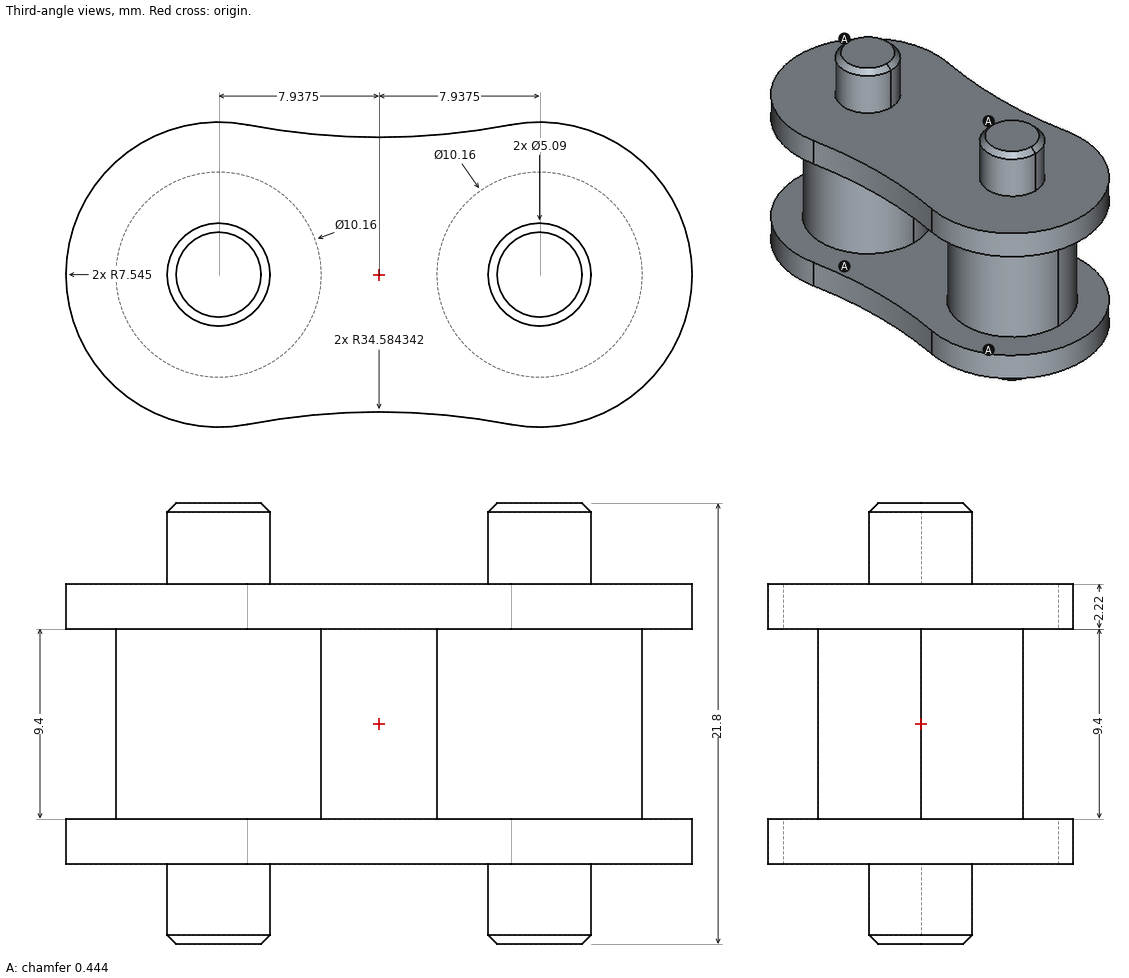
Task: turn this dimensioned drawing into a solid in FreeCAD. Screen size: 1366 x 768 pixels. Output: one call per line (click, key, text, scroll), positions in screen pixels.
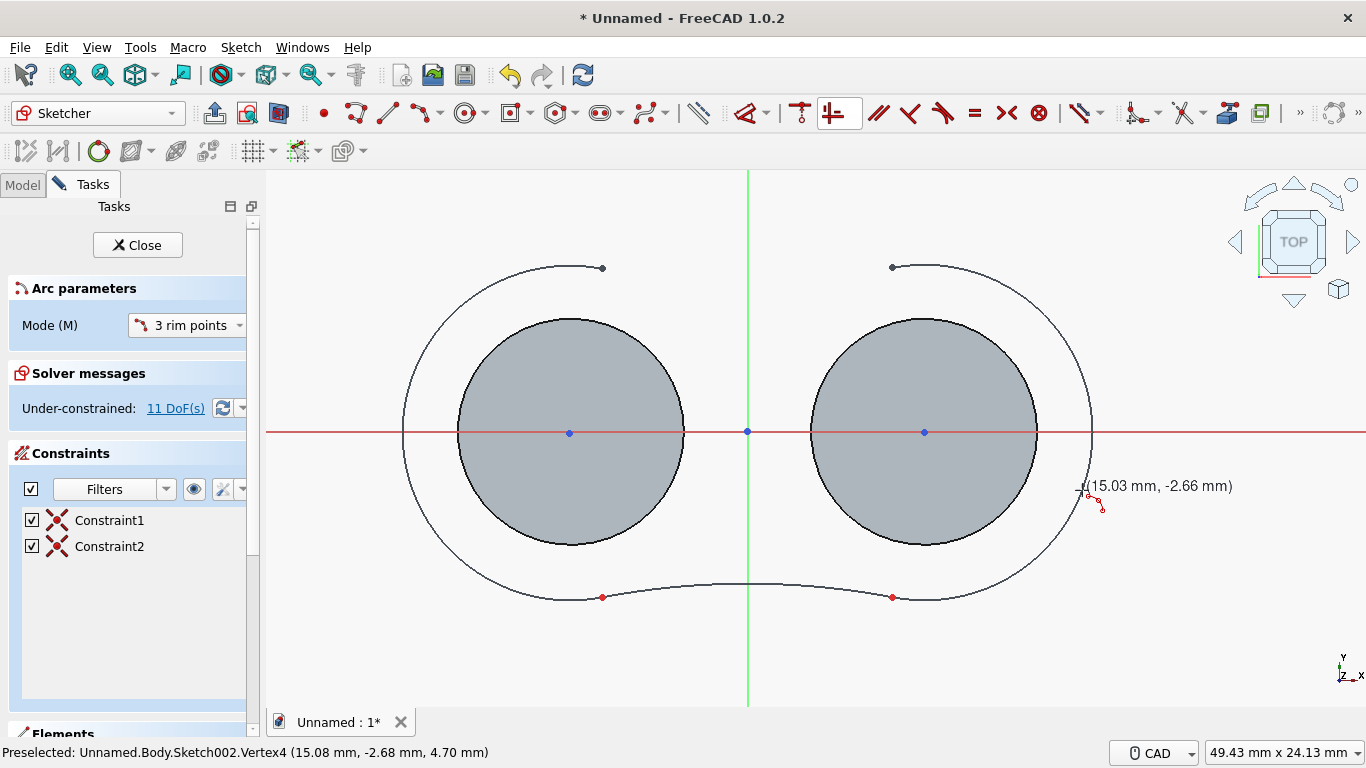
click(892, 268)
click(602, 269)
click(718, 280)
key(Escape)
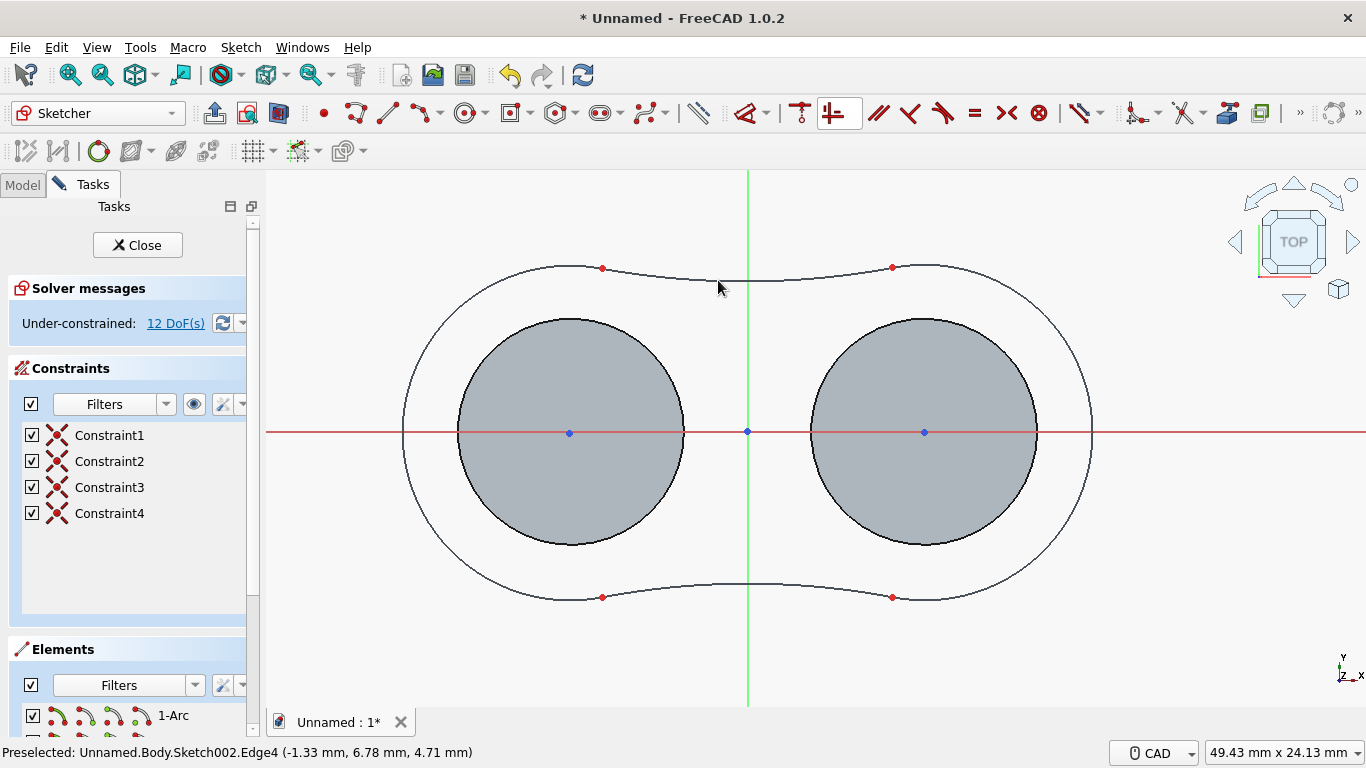
click(443, 324)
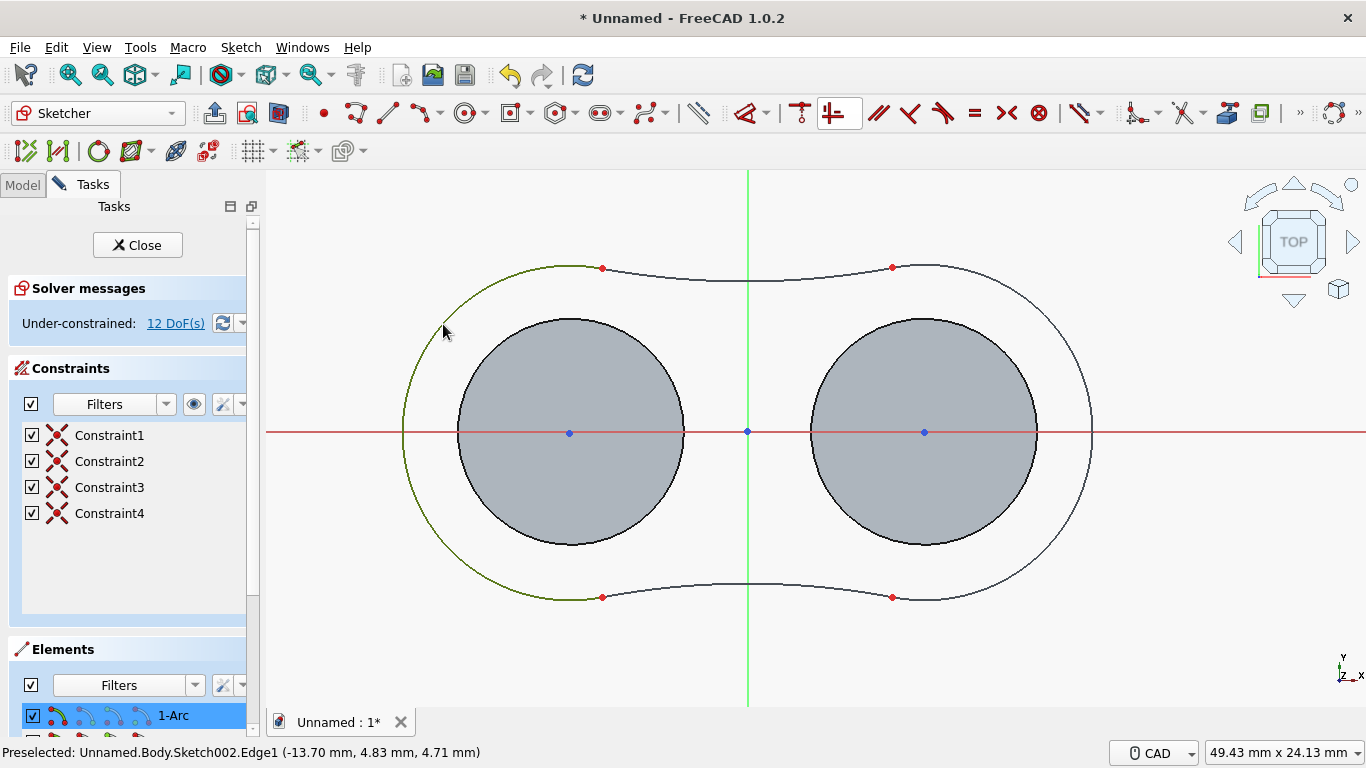
click(806, 586)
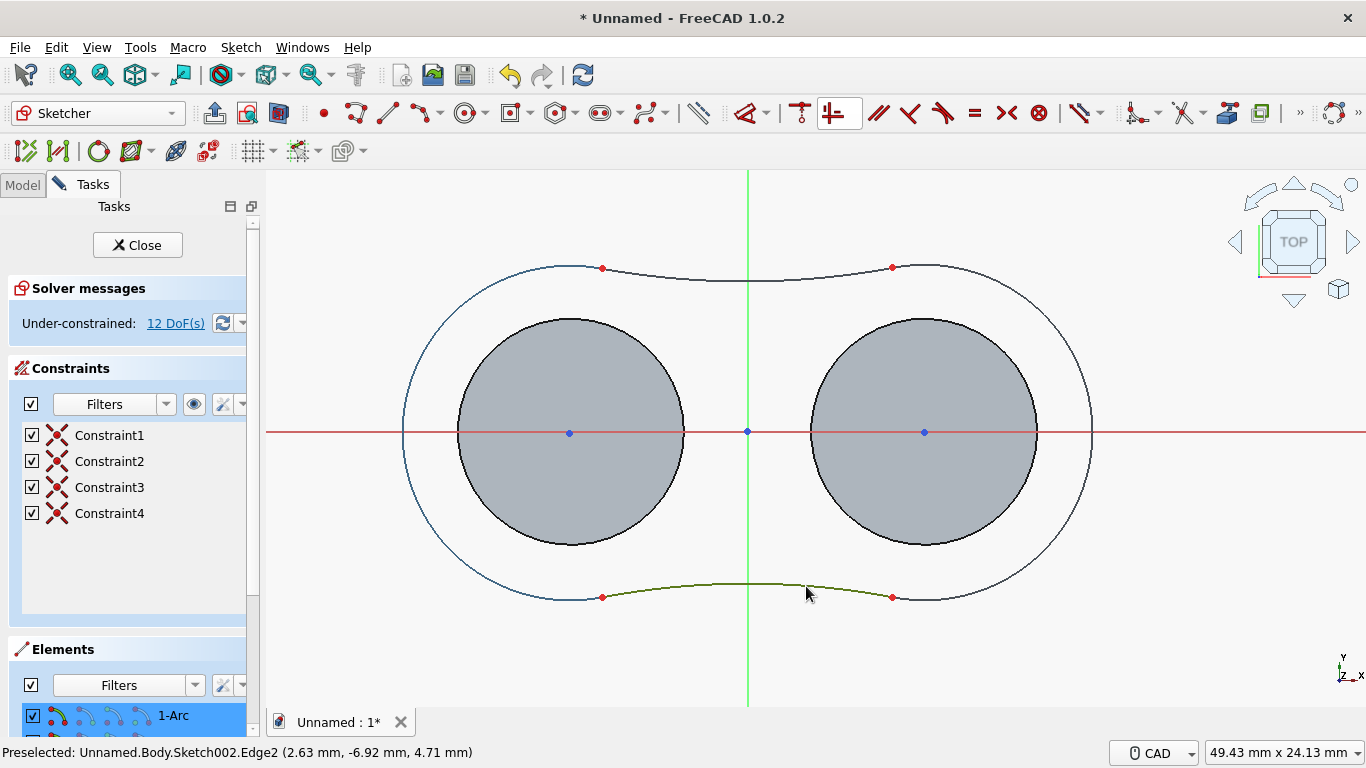
key(t)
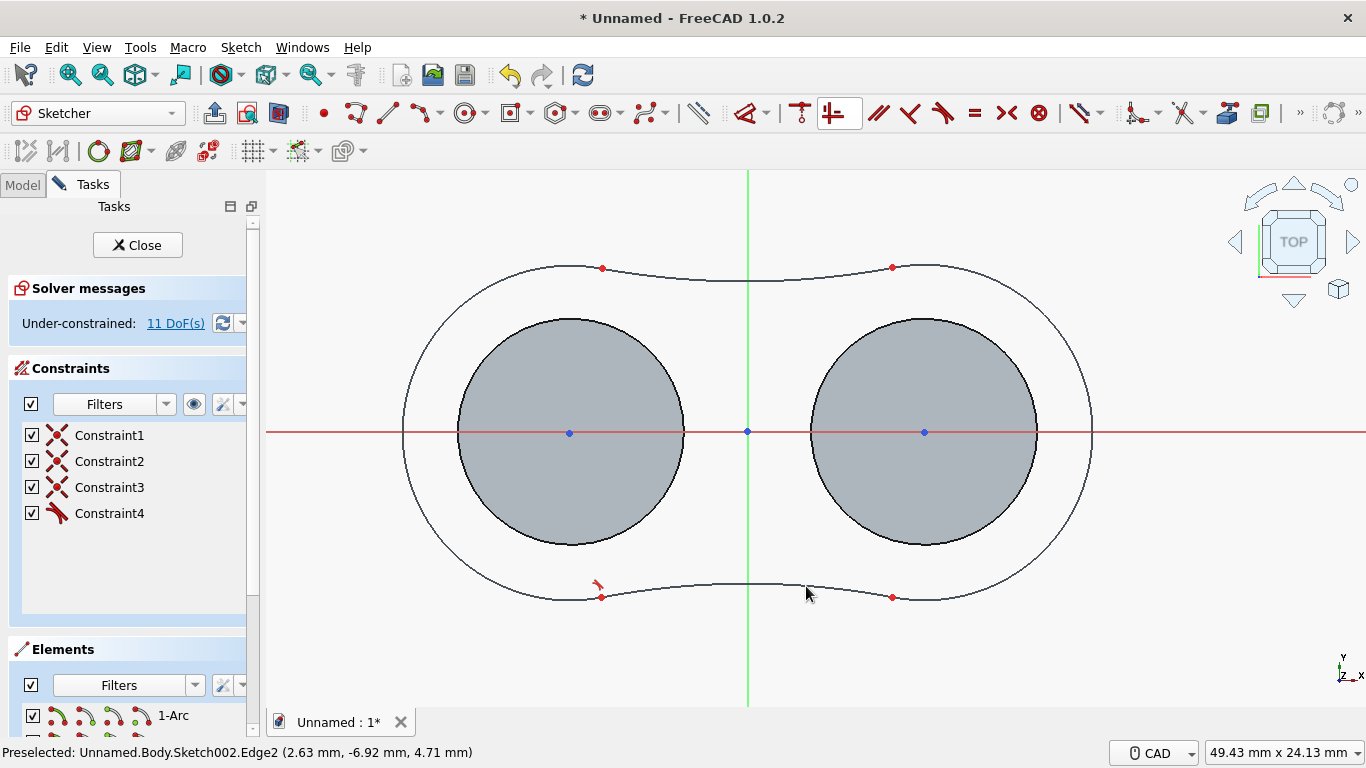
click(443, 324)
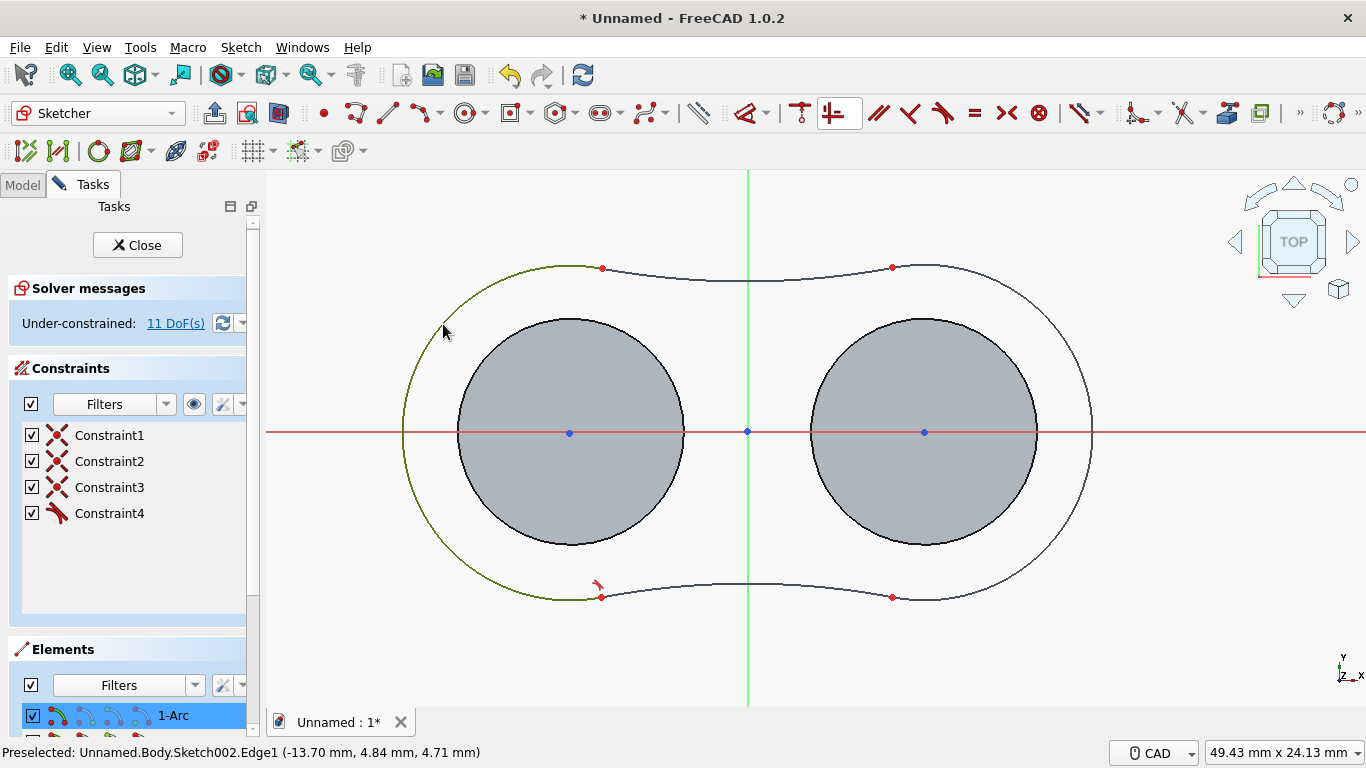
click(689, 280)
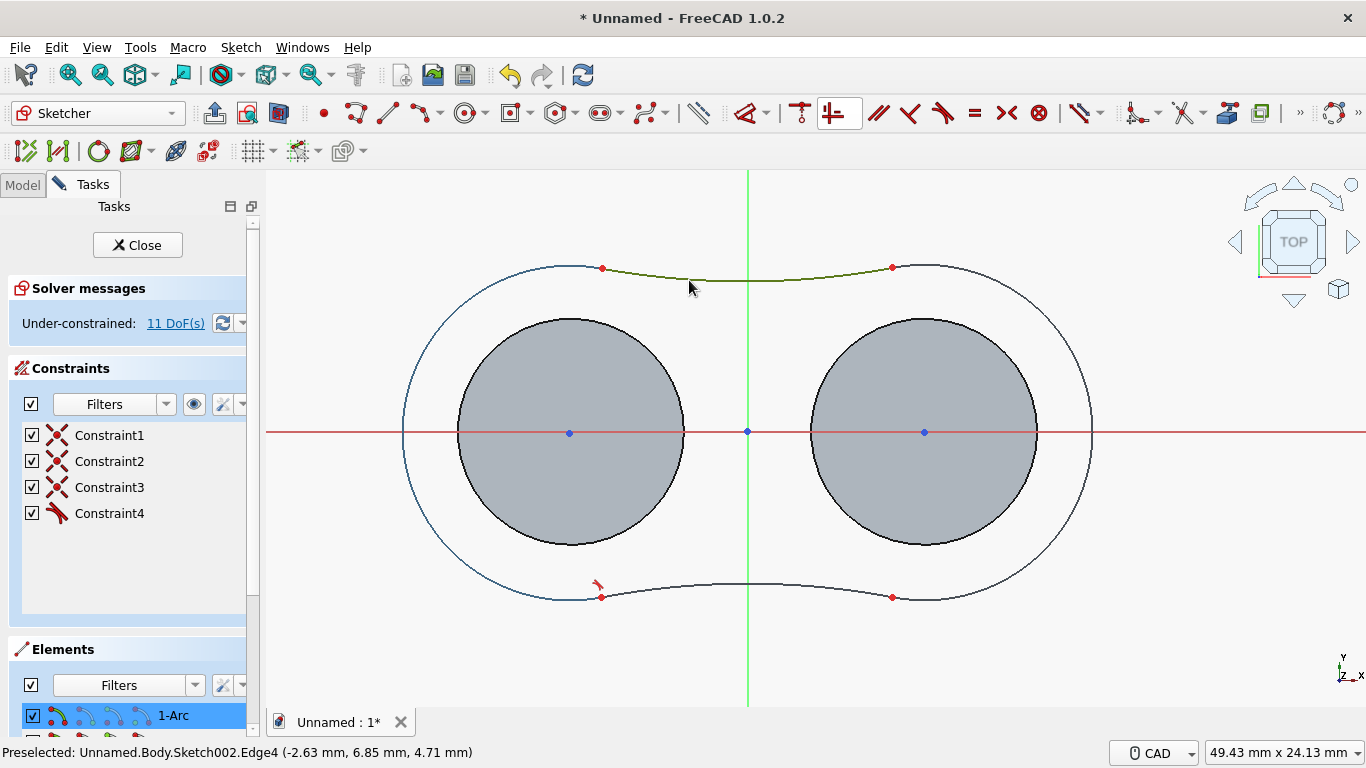
key(t)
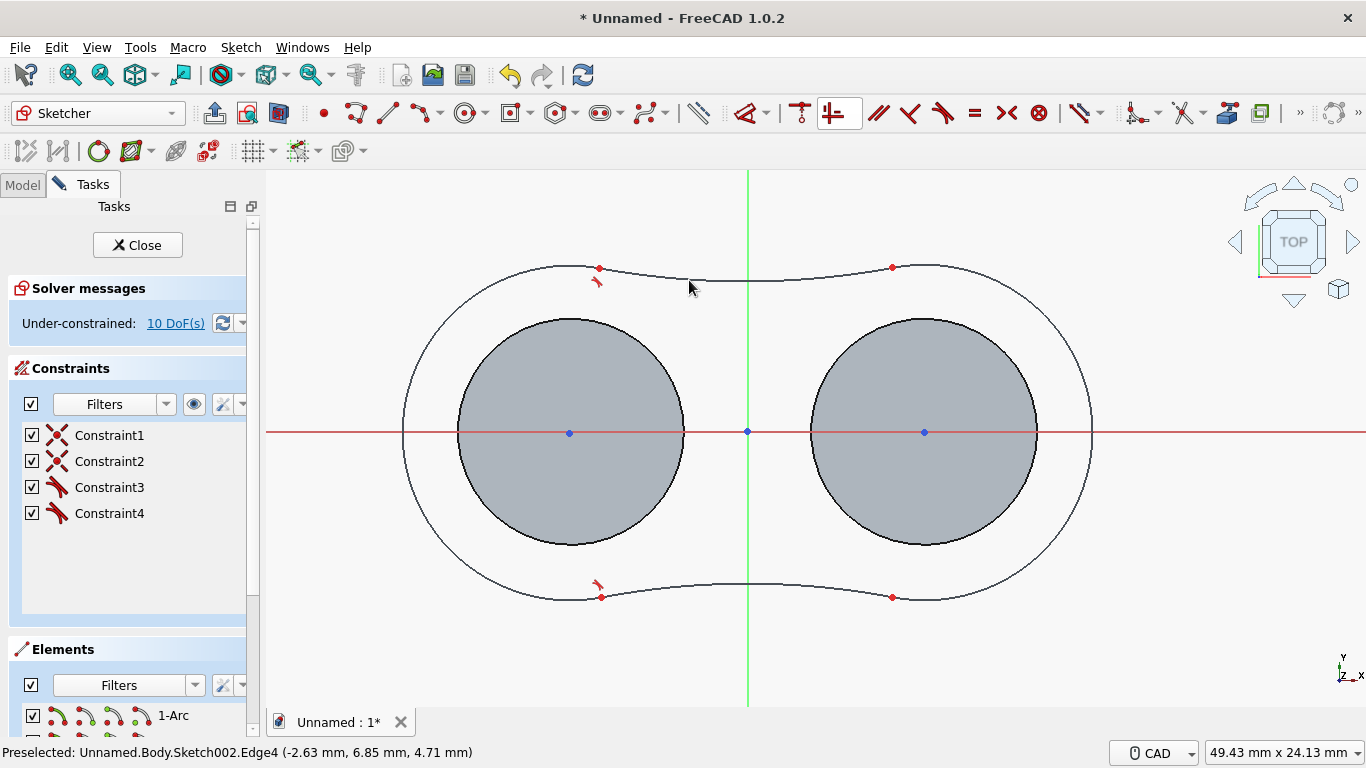
click(806, 586)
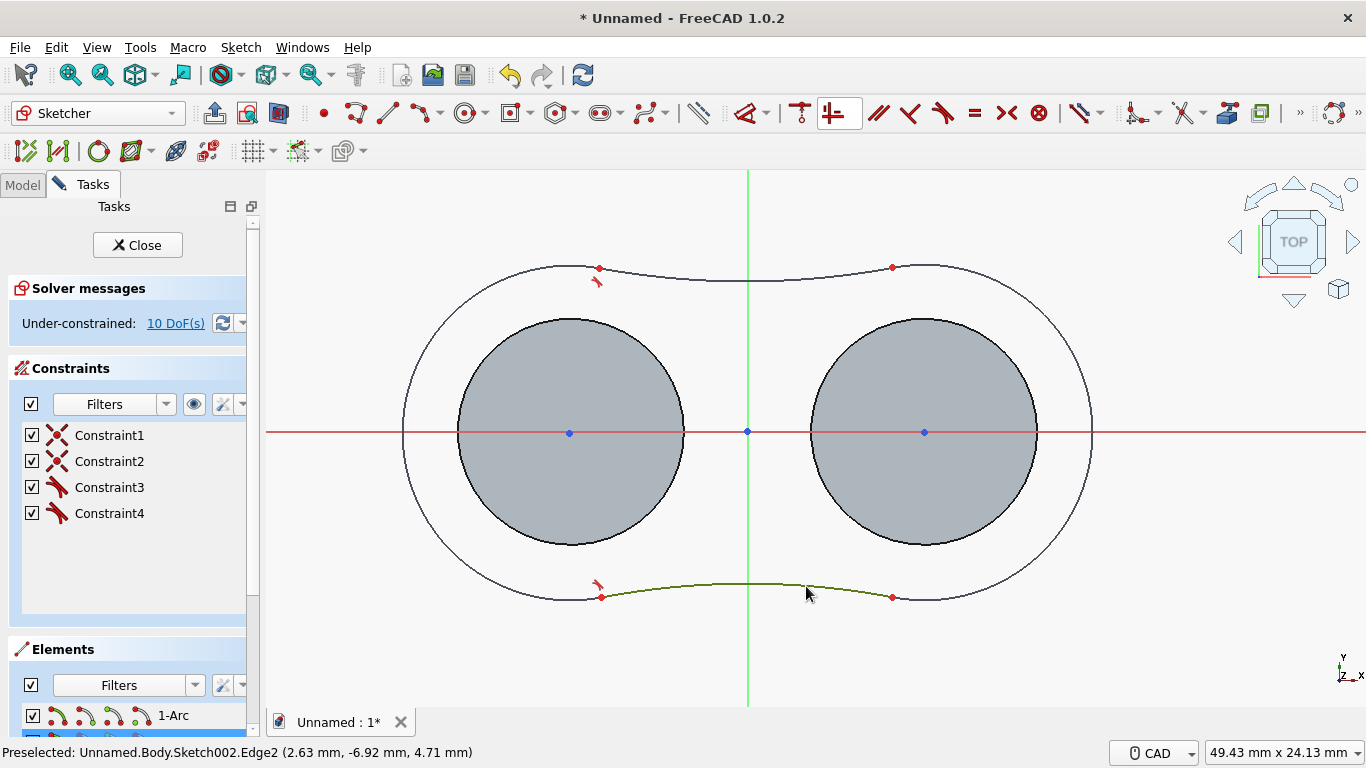
click(1053, 541)